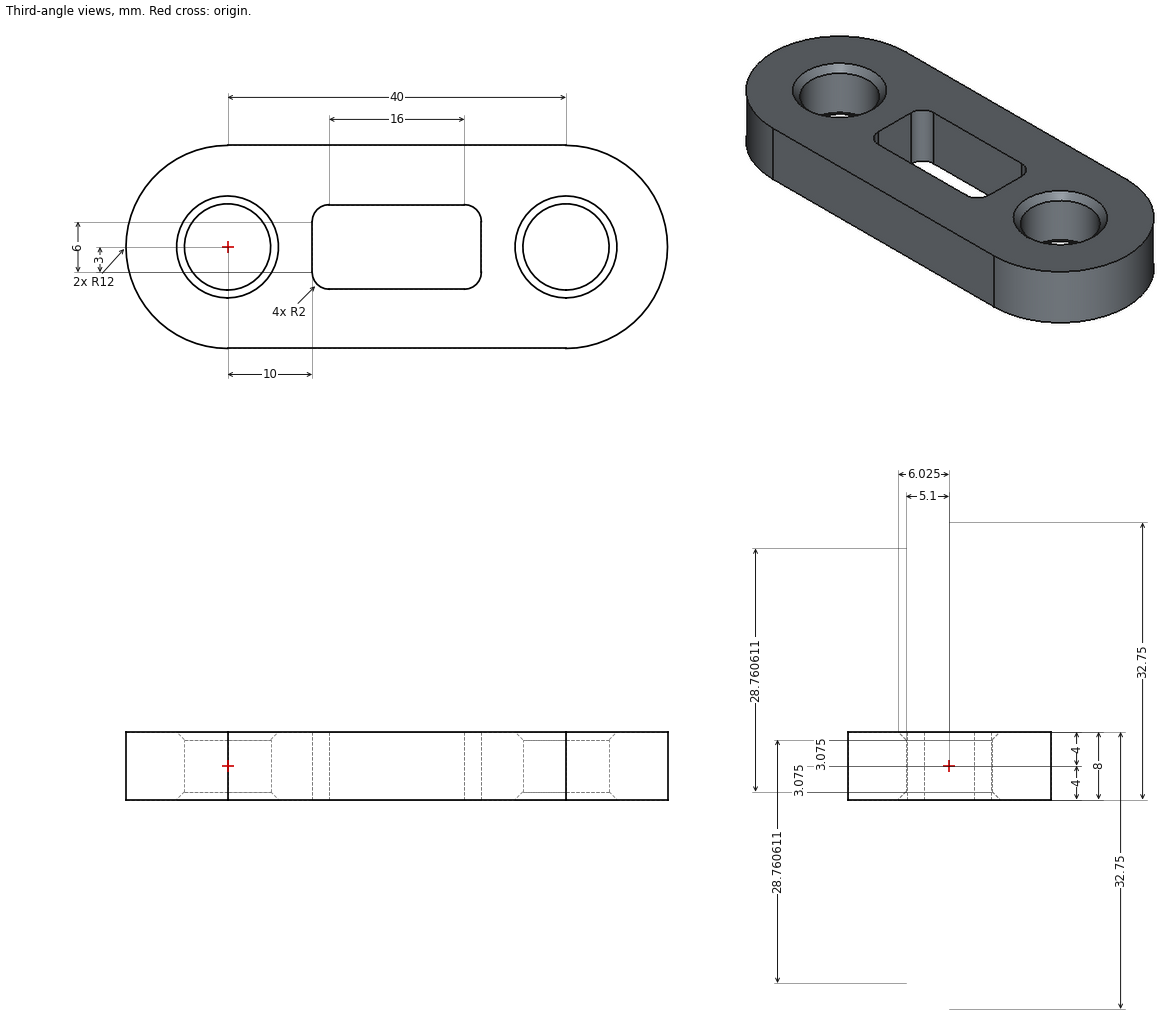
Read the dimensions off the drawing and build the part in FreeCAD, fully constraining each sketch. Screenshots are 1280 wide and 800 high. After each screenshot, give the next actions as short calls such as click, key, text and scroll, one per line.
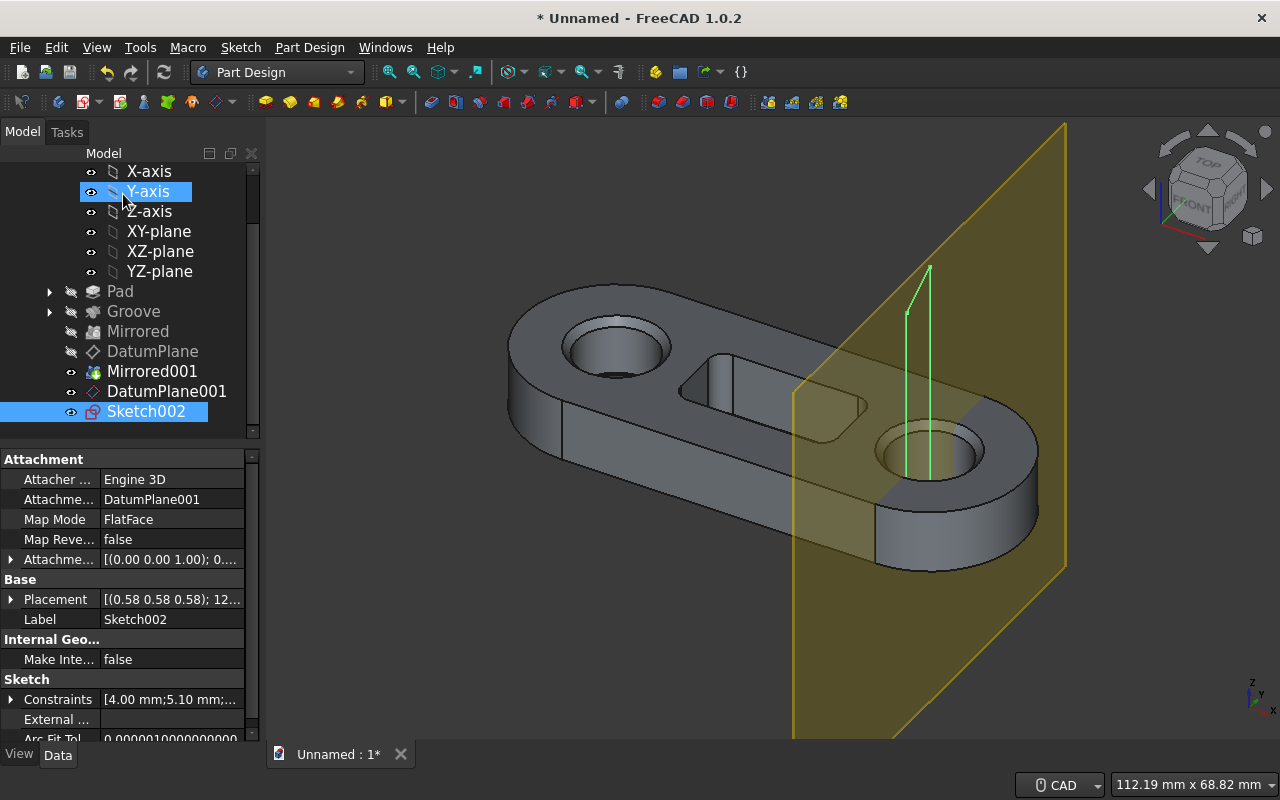
click(480, 102)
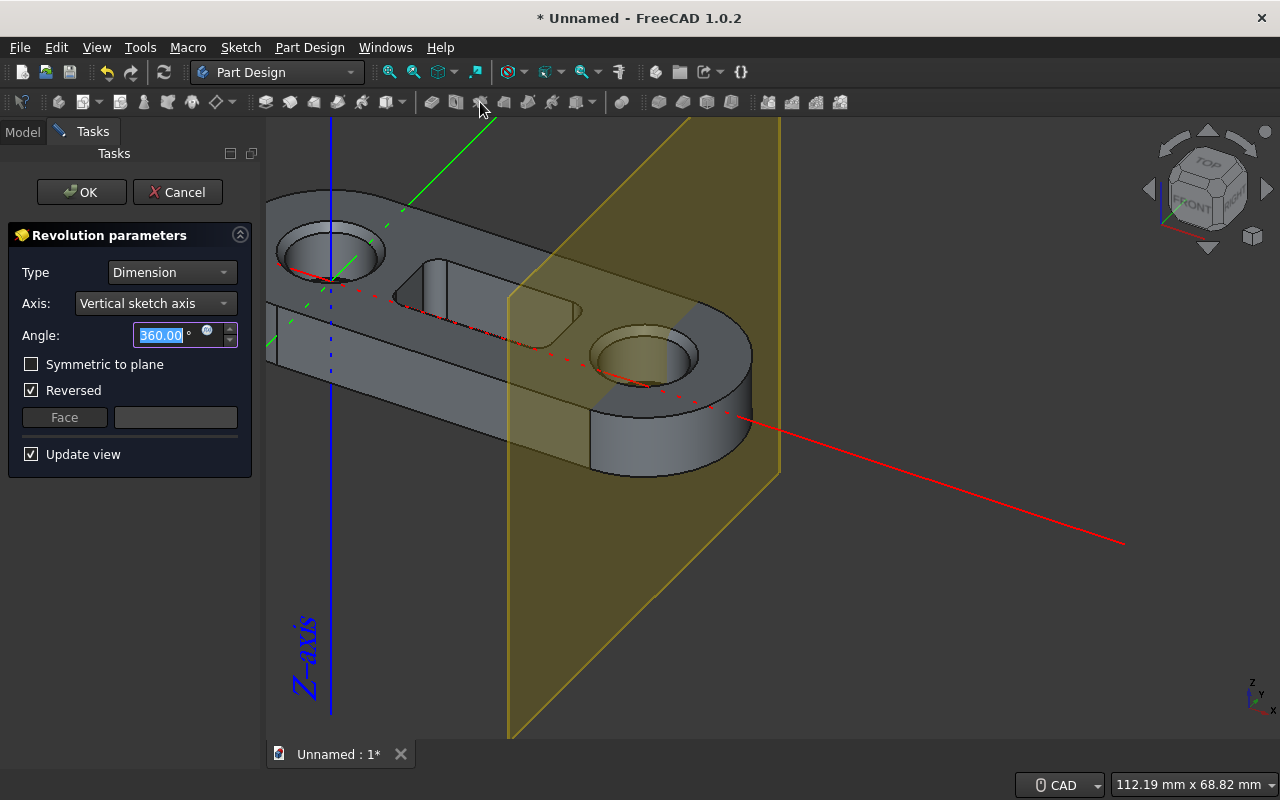
click(82, 192)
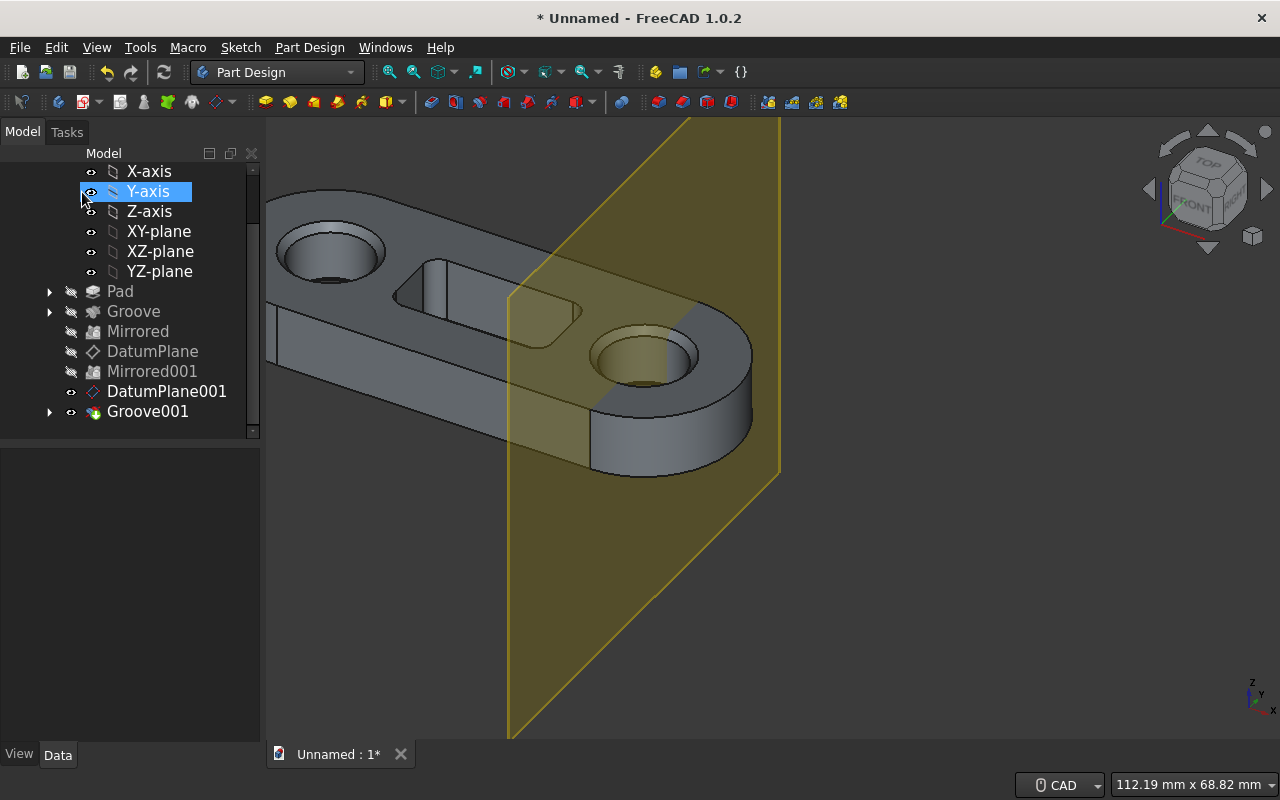
click(116, 392)
key(space)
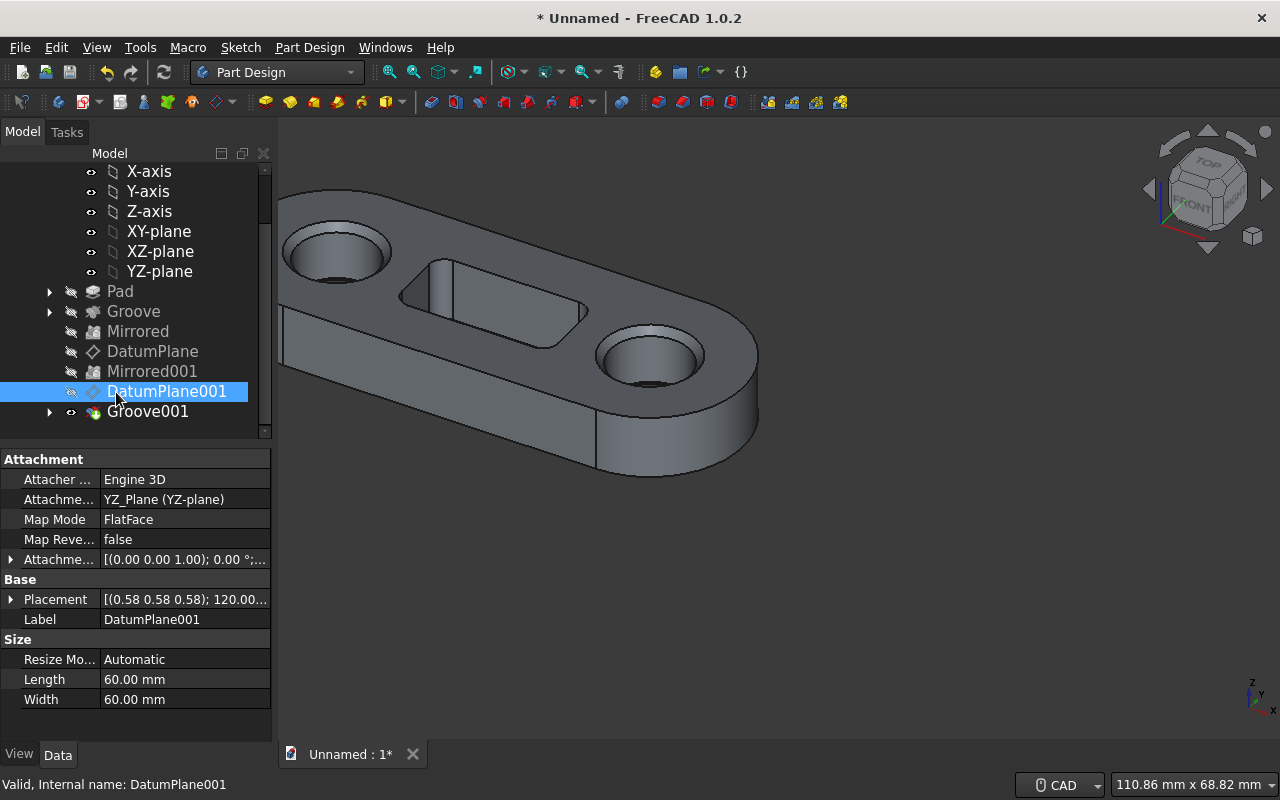
key(0)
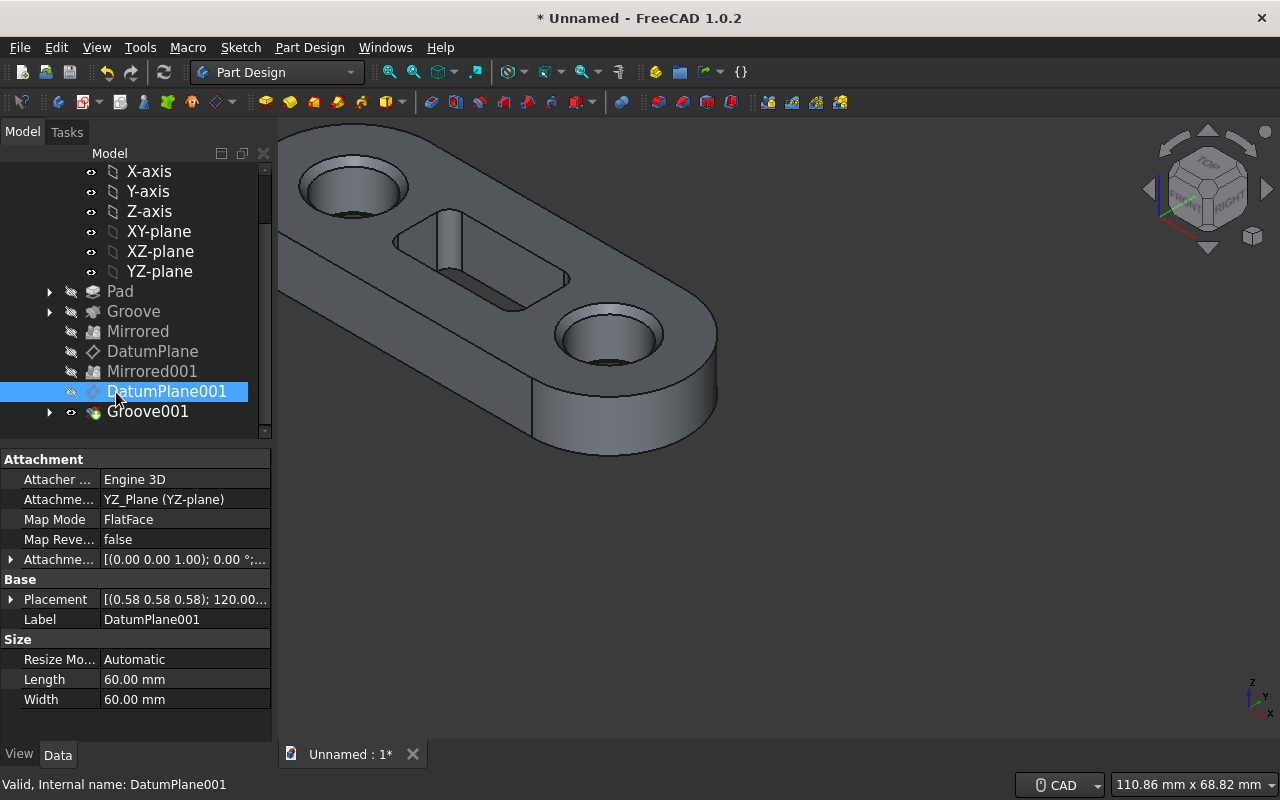
key(v)
key(f)